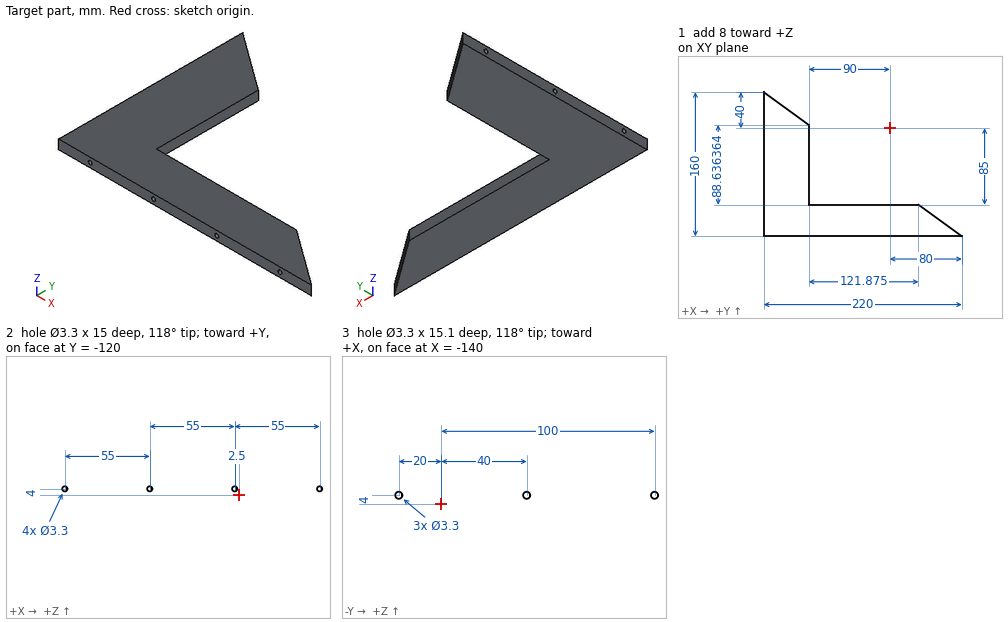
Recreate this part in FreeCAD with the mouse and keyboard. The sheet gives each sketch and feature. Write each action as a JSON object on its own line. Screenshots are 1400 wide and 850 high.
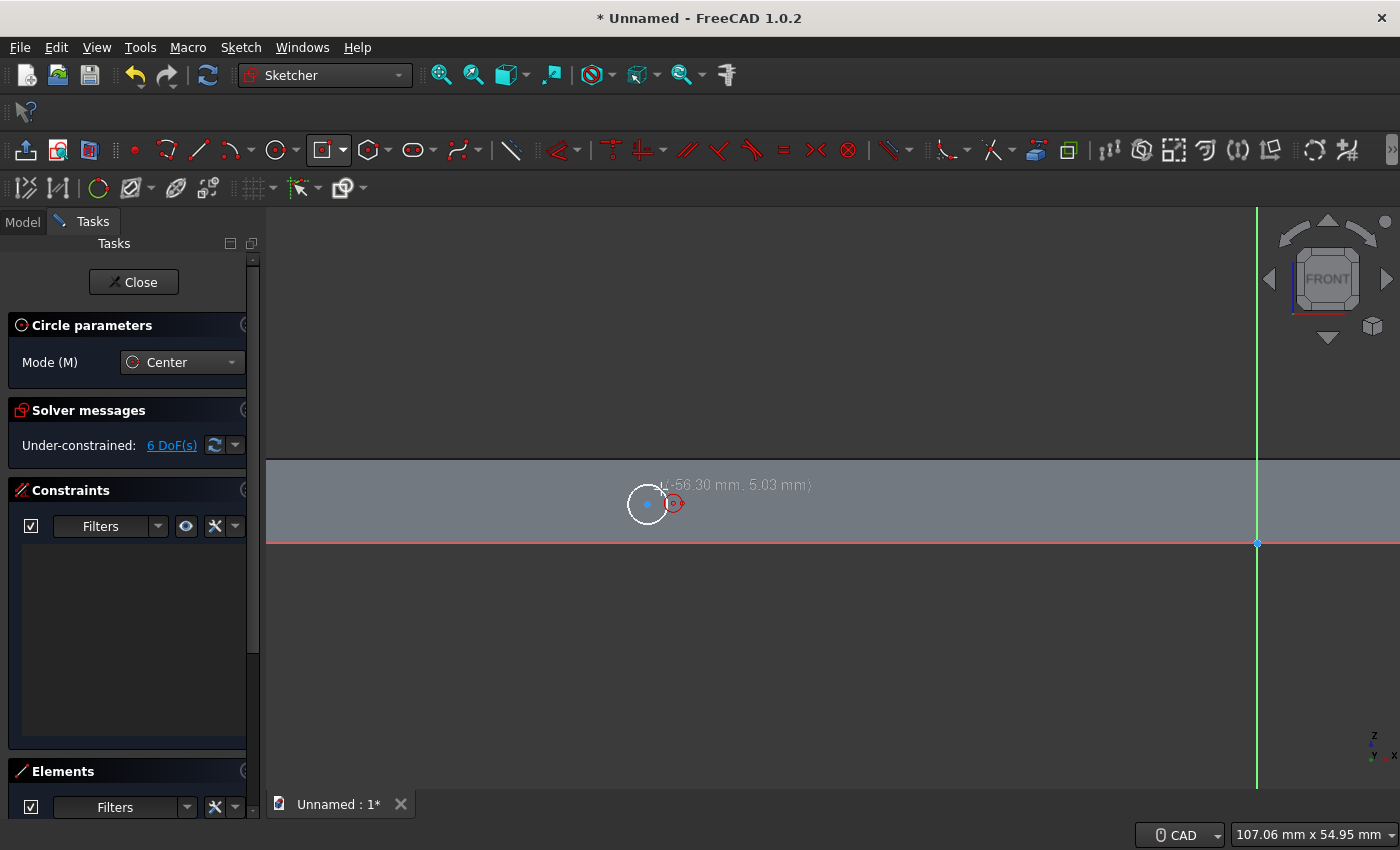
{"action": "scroll", "coordinate": [1231, 501], "scroll_direction": "up", "scroll_amount": 2}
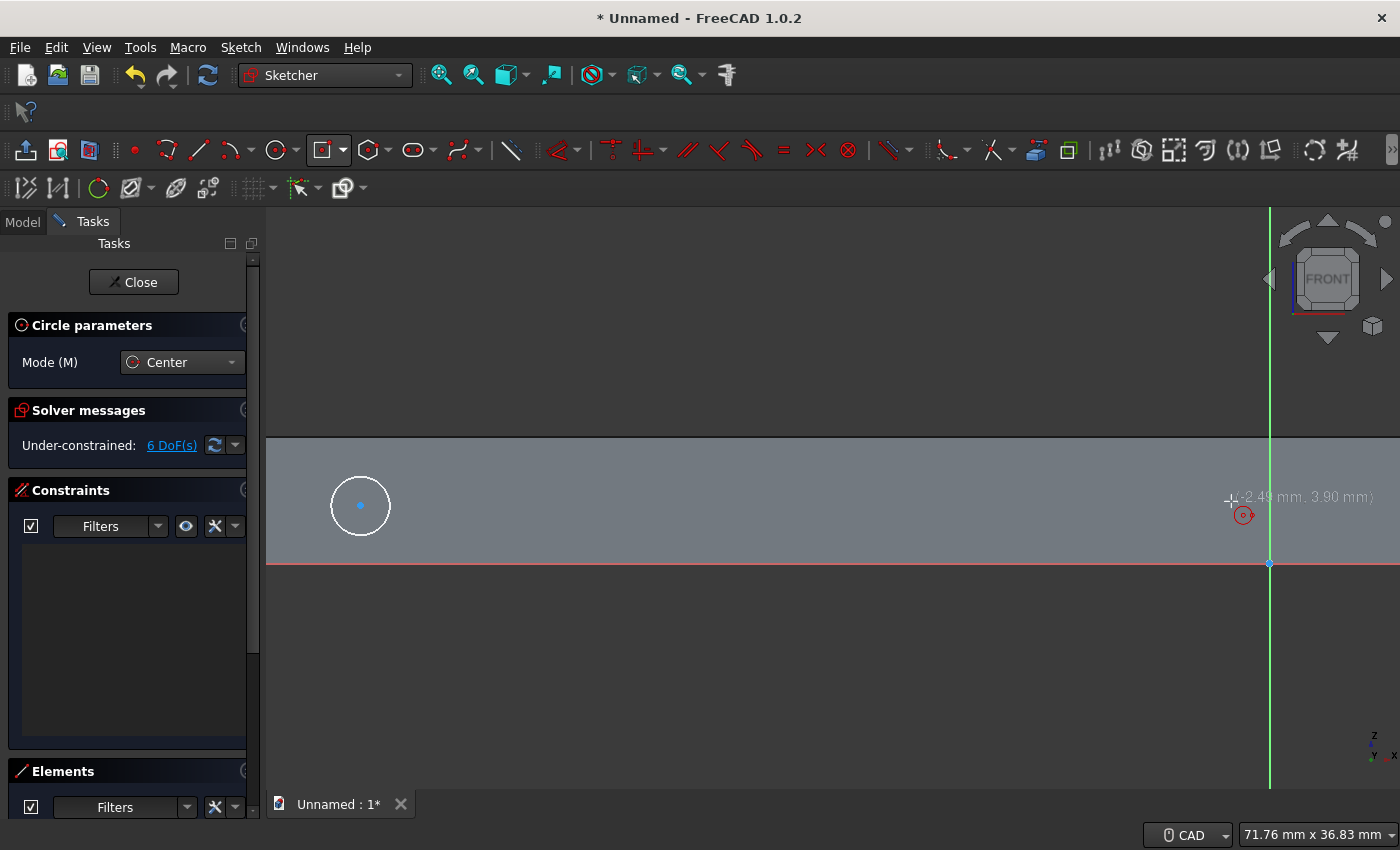
{"action": "left_click", "coordinate": [1230, 501]}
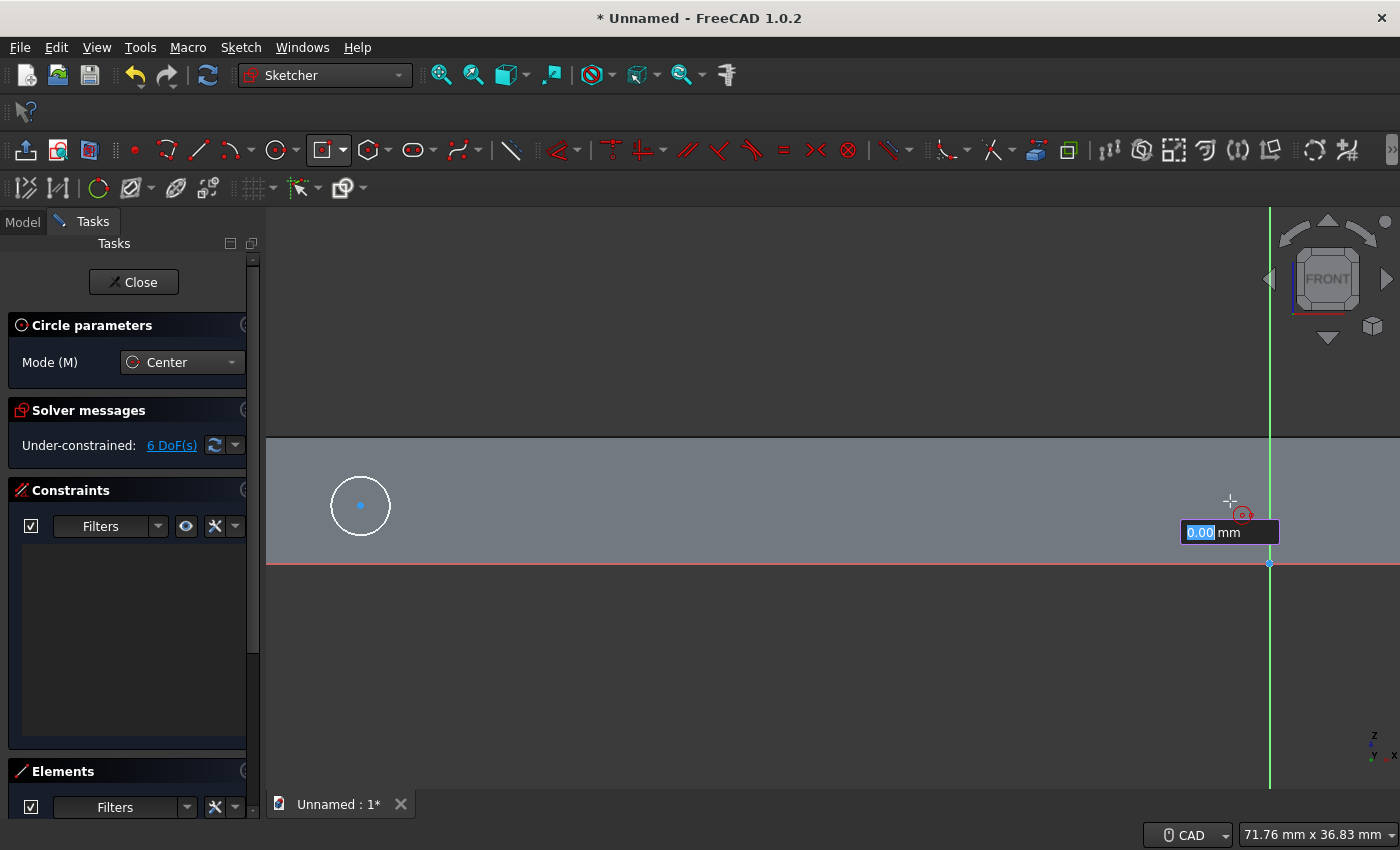
{"action": "scroll", "coordinate": [754, 491], "scroll_direction": "down", "scroll_amount": 7}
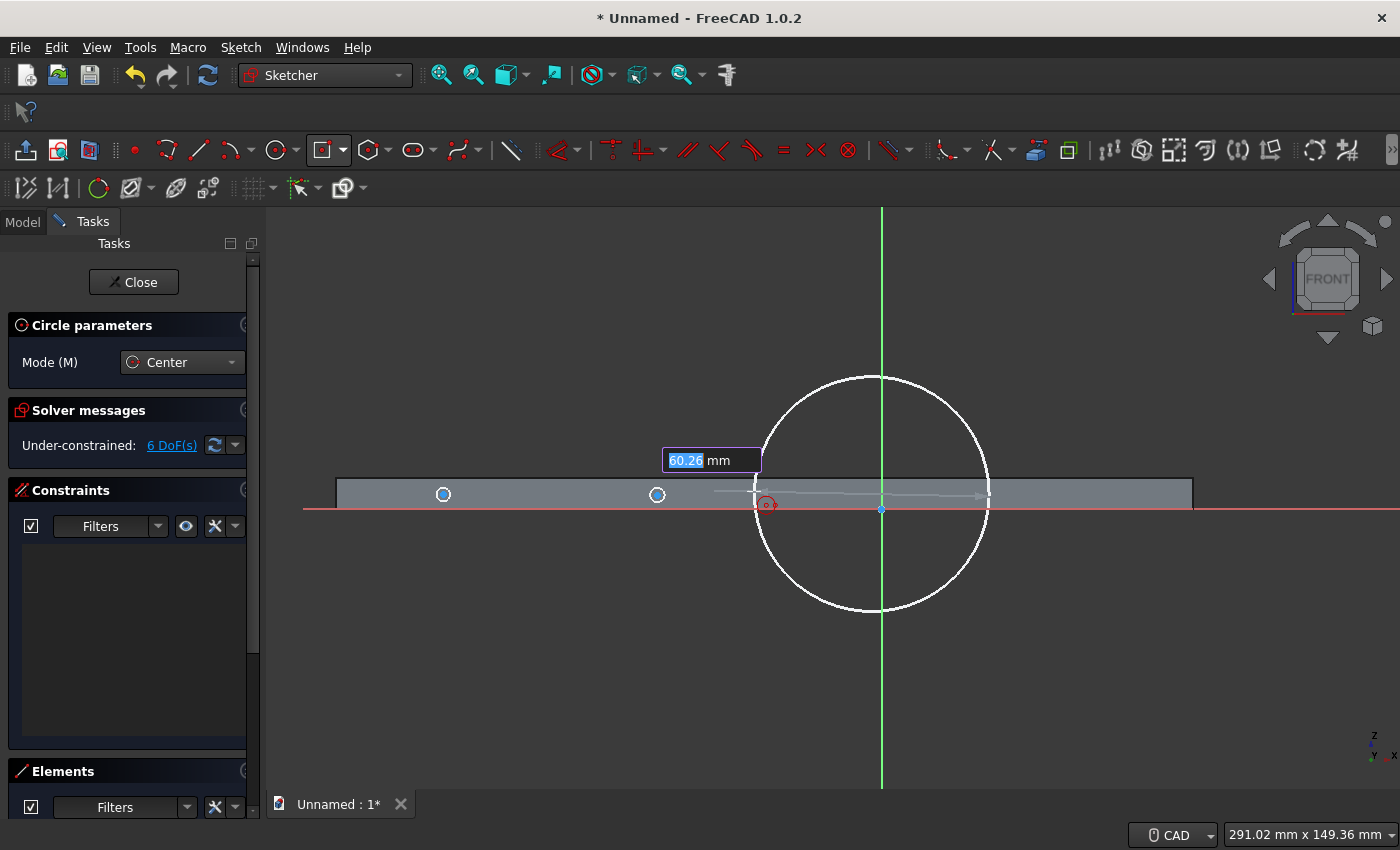
{"action": "scroll", "coordinate": [876, 489], "scroll_direction": "up", "scroll_amount": 6}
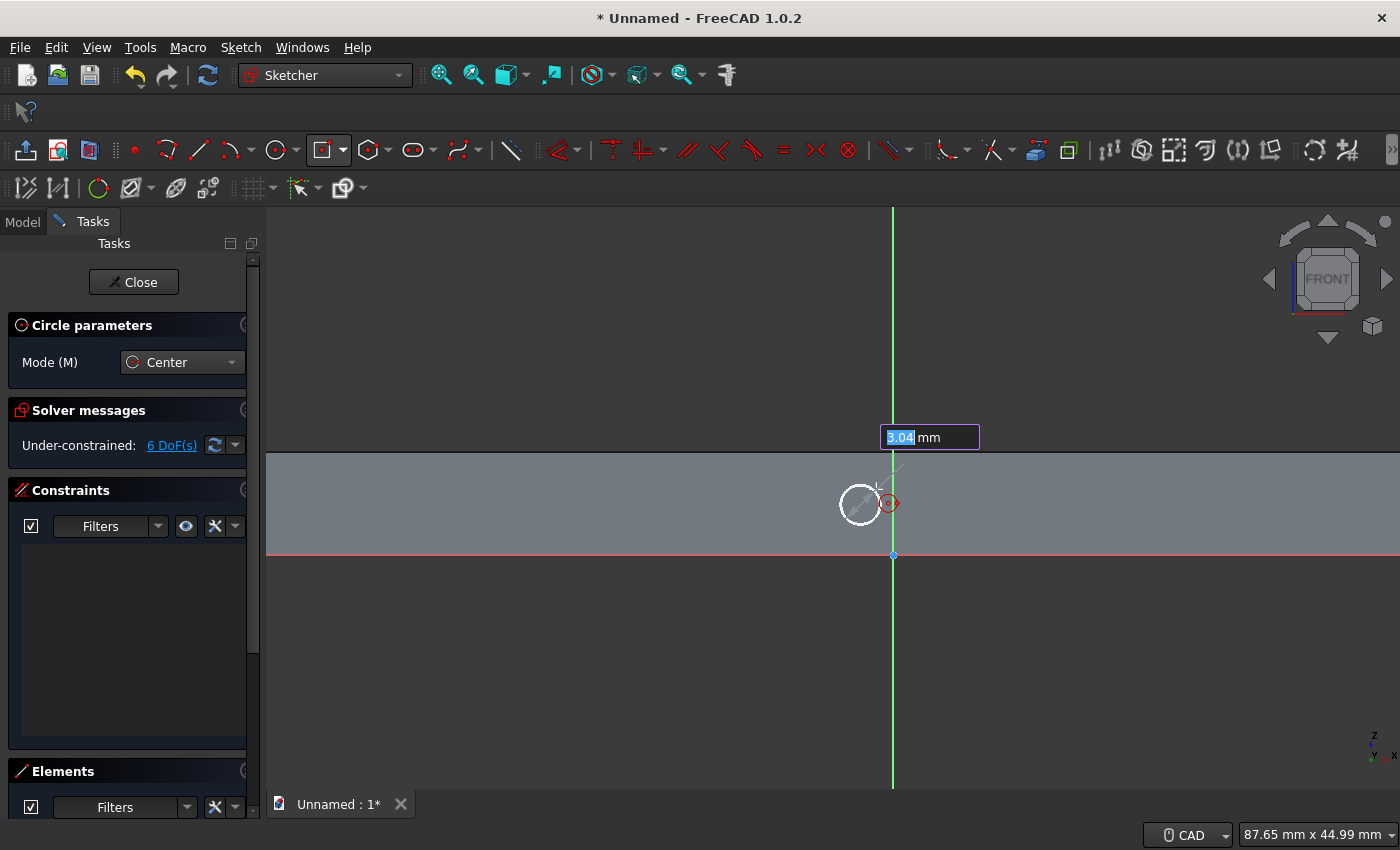
{"action": "left_click", "coordinate": [876, 489]}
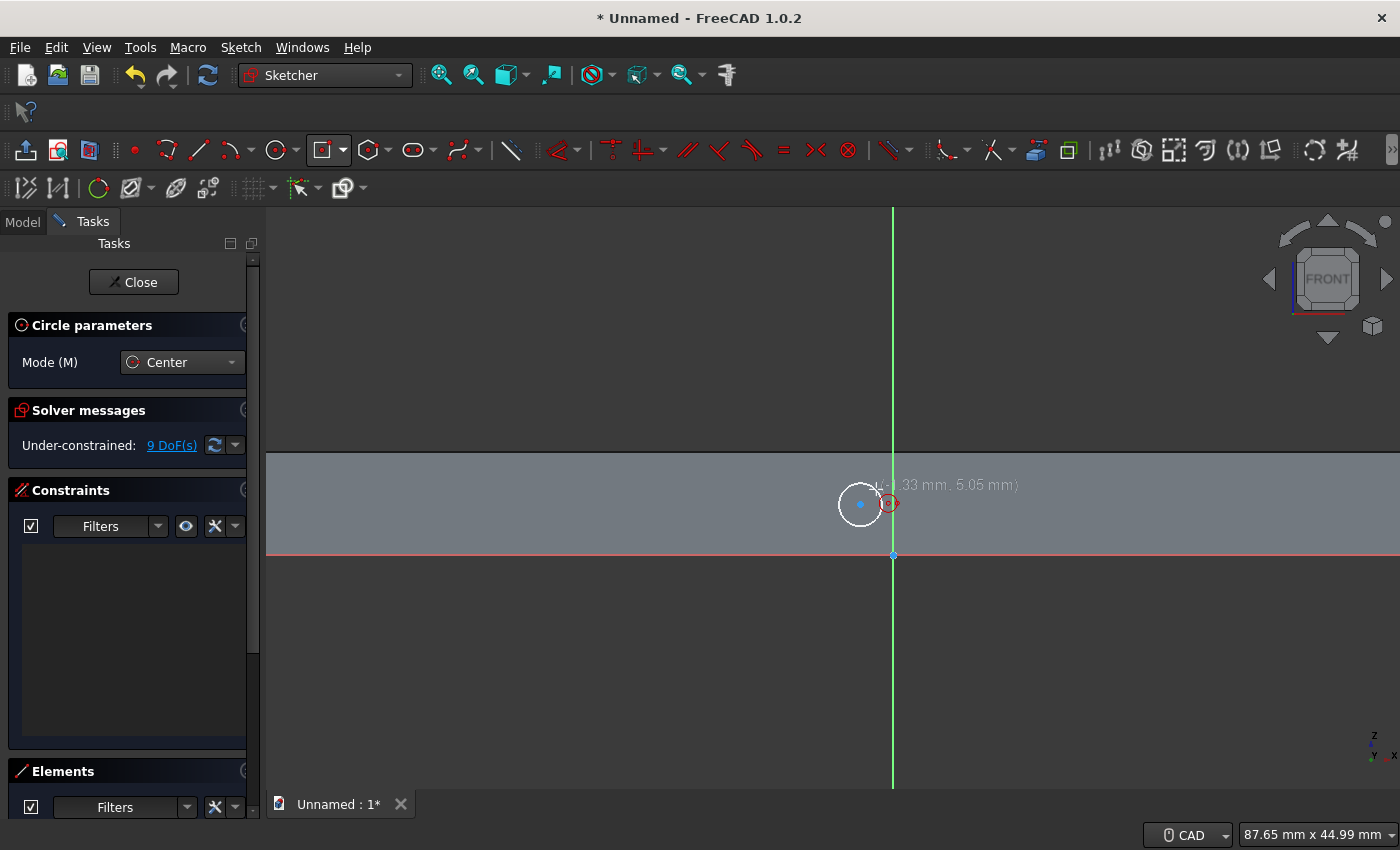
{"action": "scroll", "coordinate": [876, 489], "scroll_direction": "down", "scroll_amount": 6}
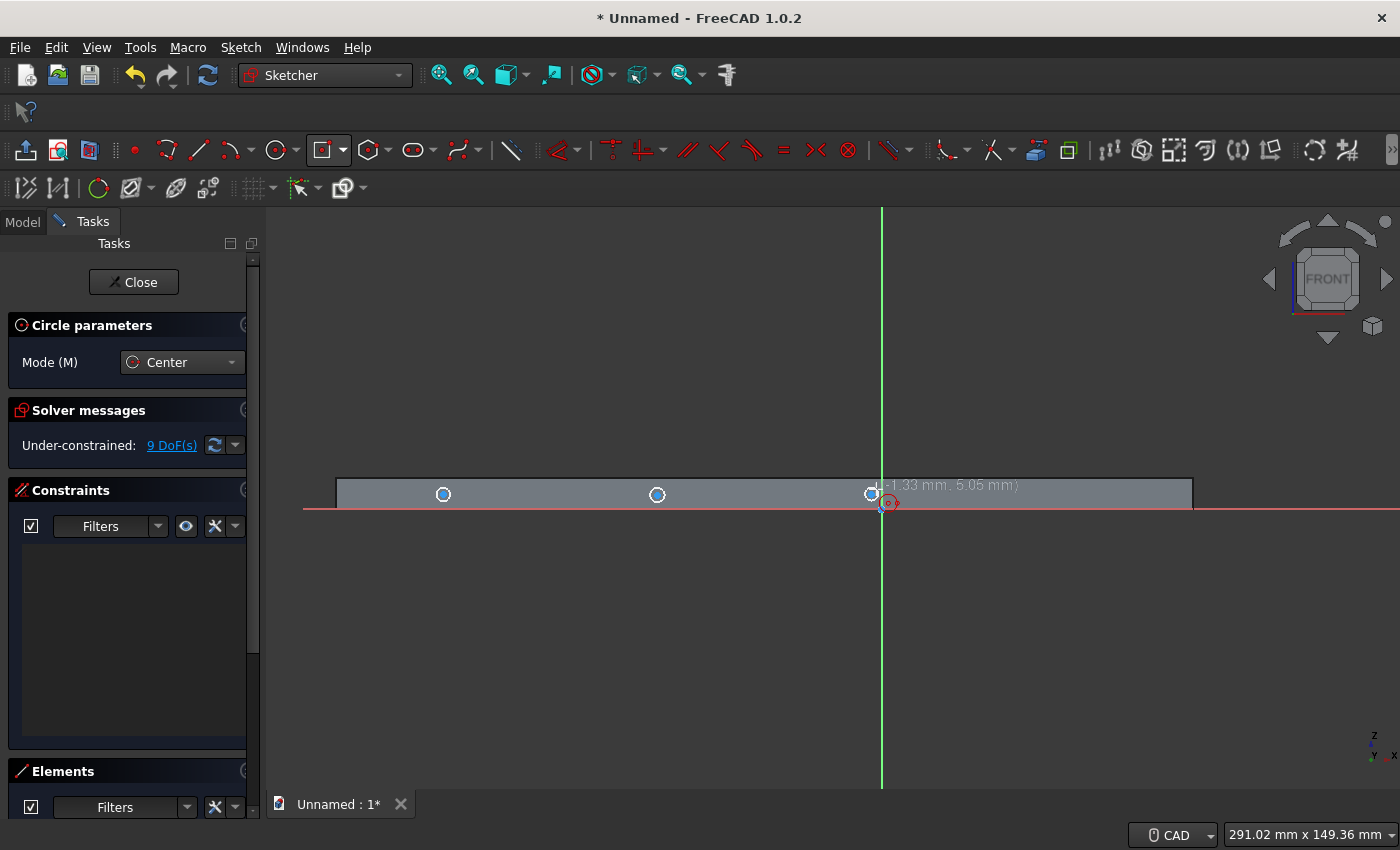
{"action": "scroll", "coordinate": [1086, 494], "scroll_direction": "up", "scroll_amount": 7}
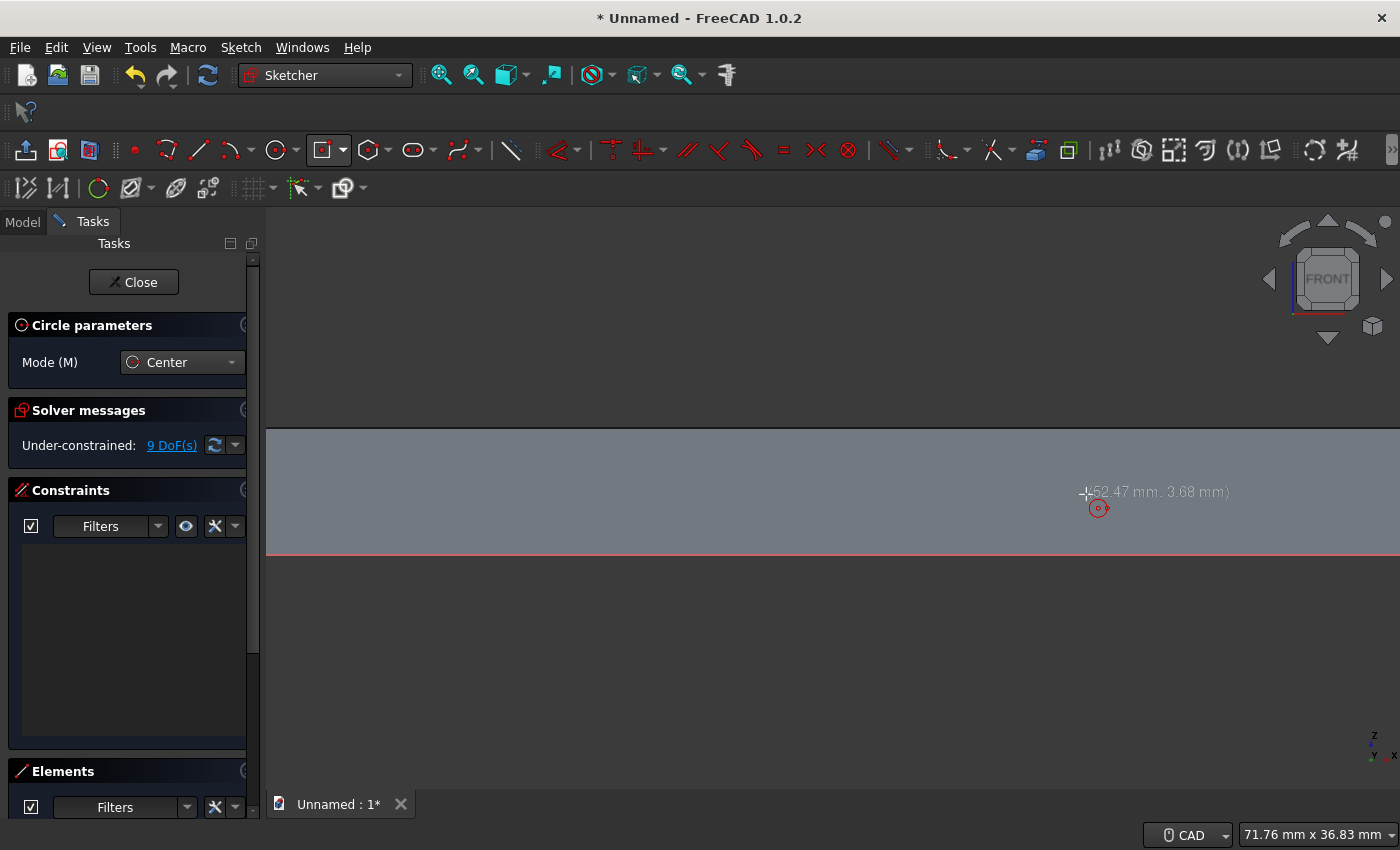
{"action": "scroll", "coordinate": [1087, 494], "scroll_direction": "down", "scroll_amount": 7}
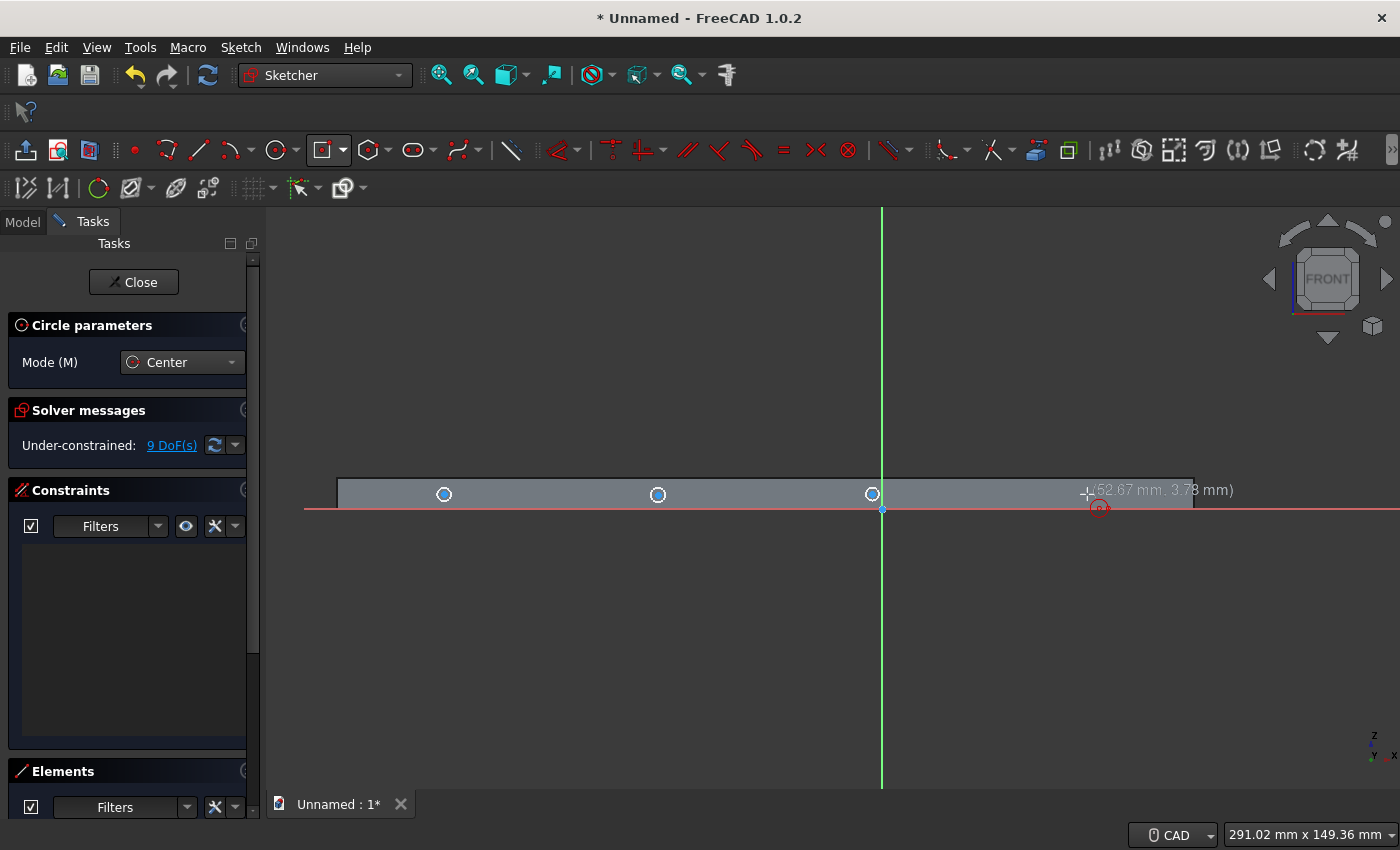
{"action": "left_click", "coordinate": [1087, 494]}